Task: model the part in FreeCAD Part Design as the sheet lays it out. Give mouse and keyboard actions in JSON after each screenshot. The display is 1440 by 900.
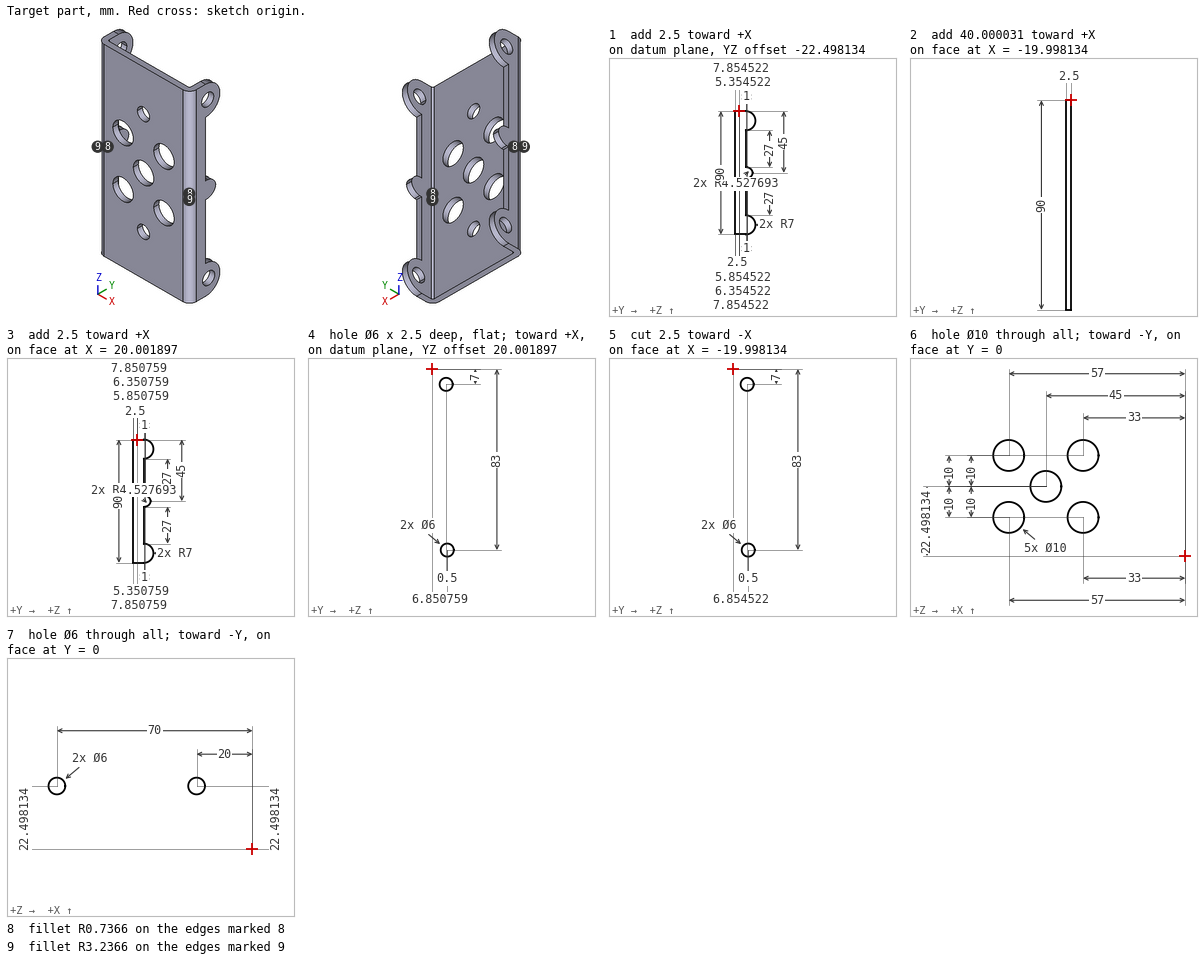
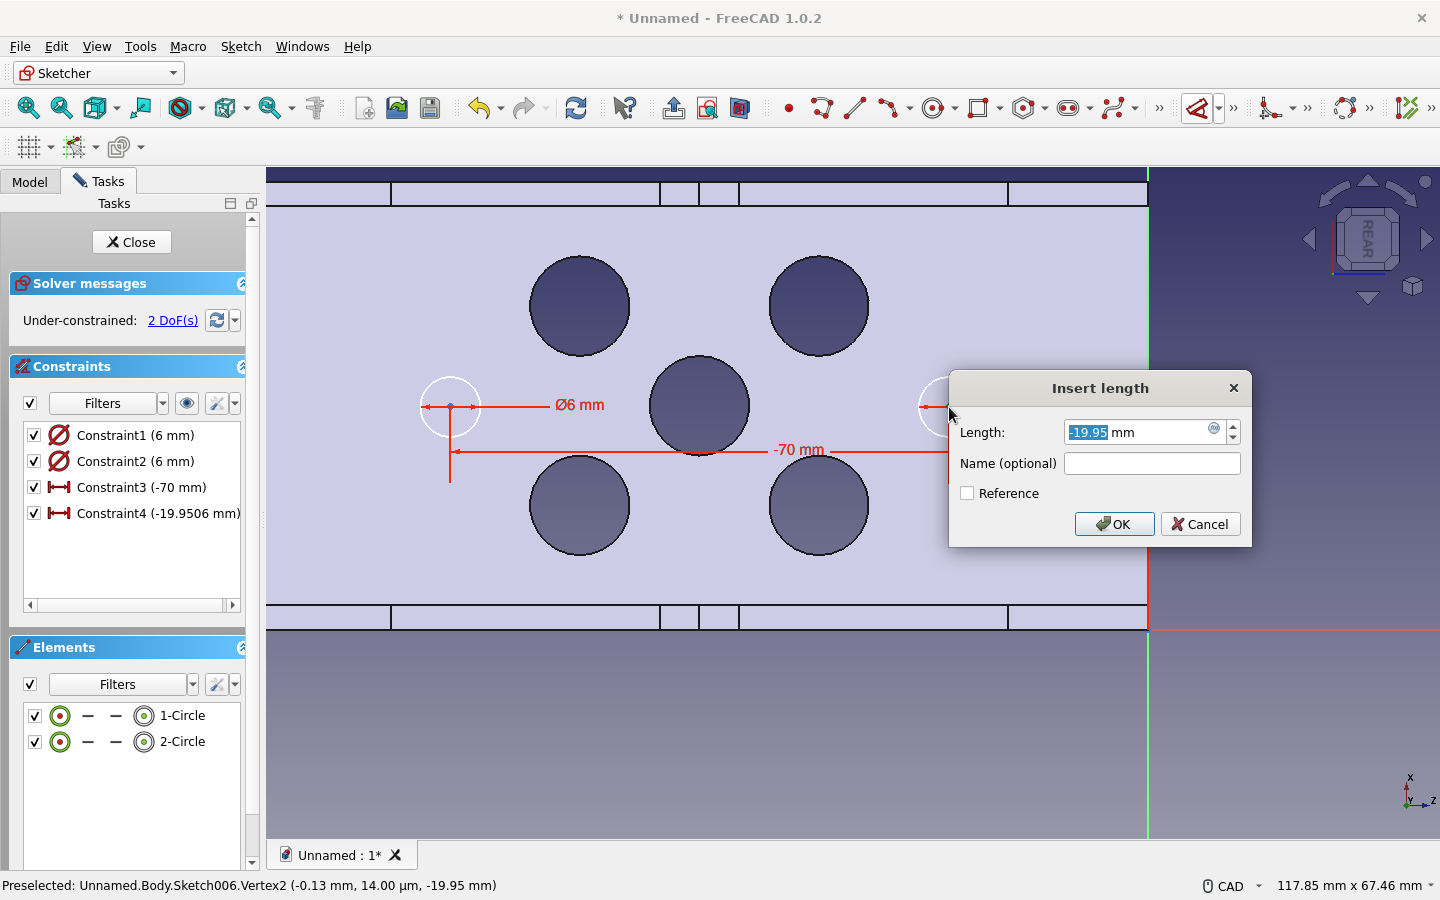
{"action": "type", "text": "-20"}
{"action": "key", "text": "Return"}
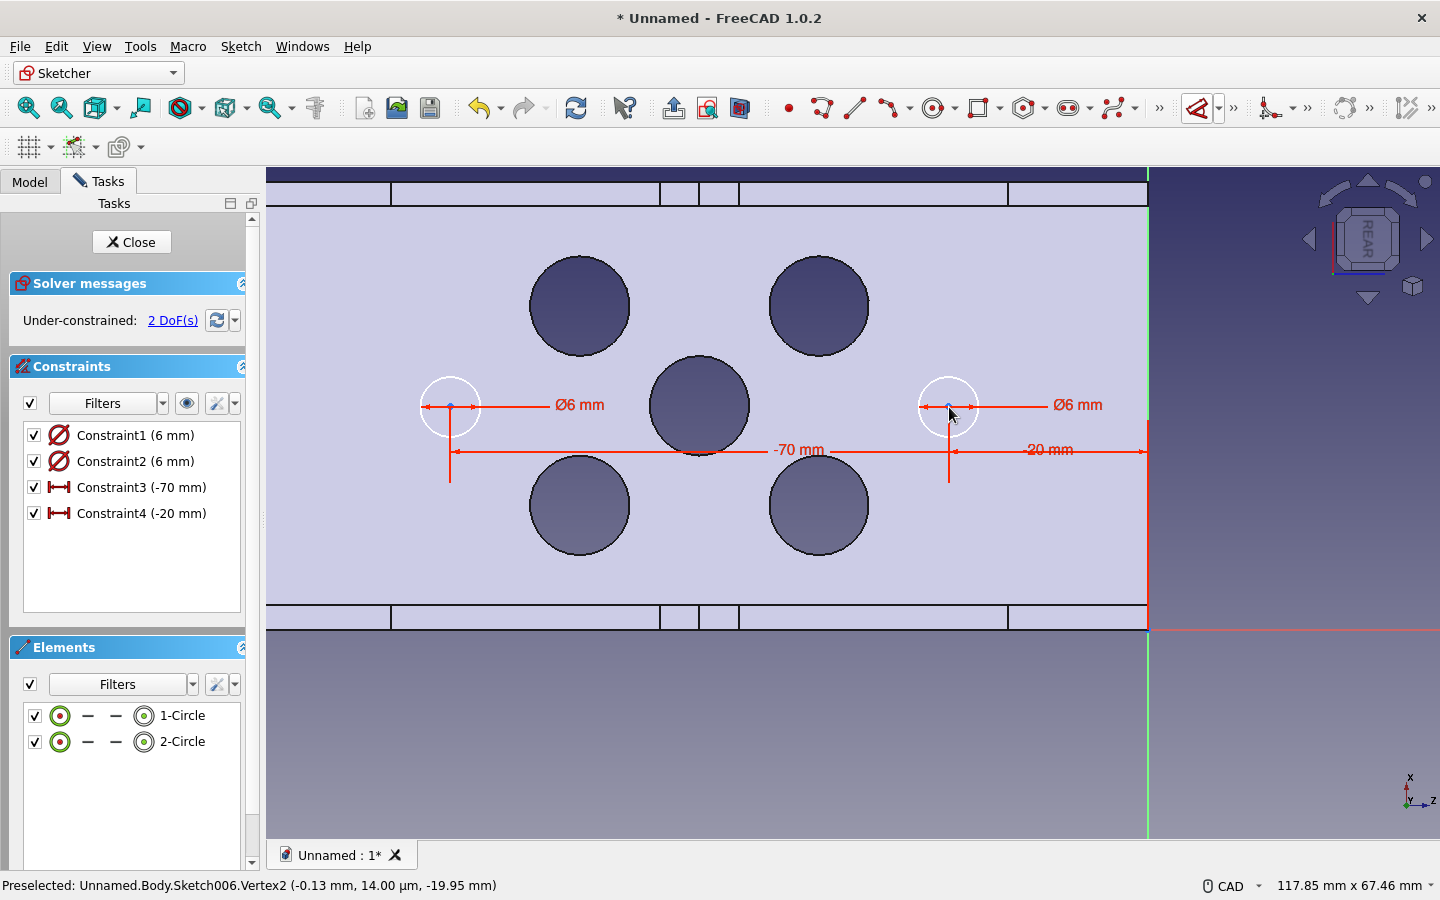
{"action": "left_click", "coordinate": [450, 407]}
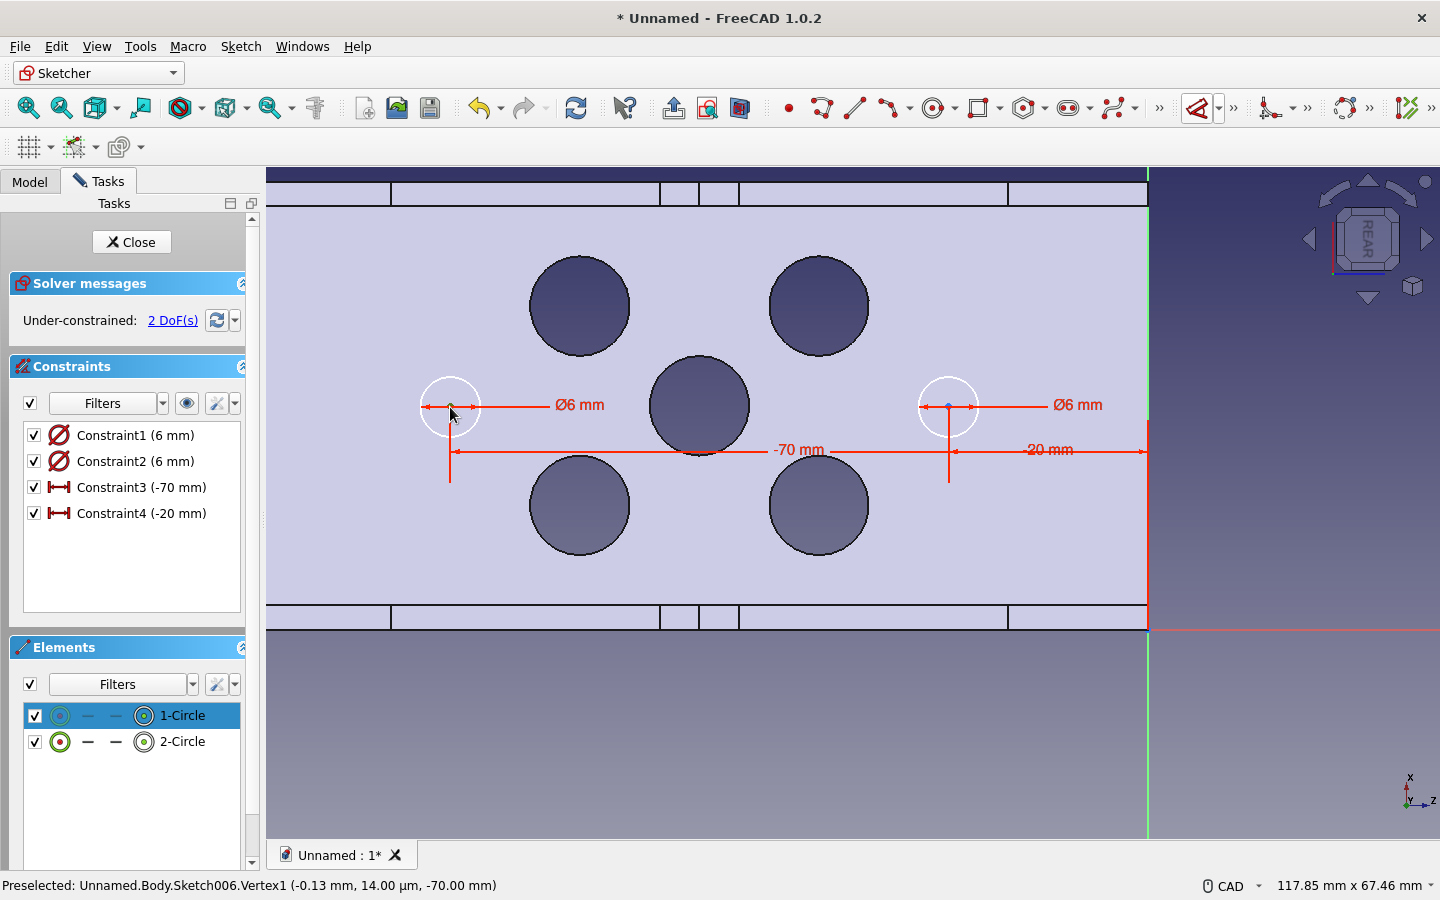
{"action": "left_click", "coordinate": [1218, 108]}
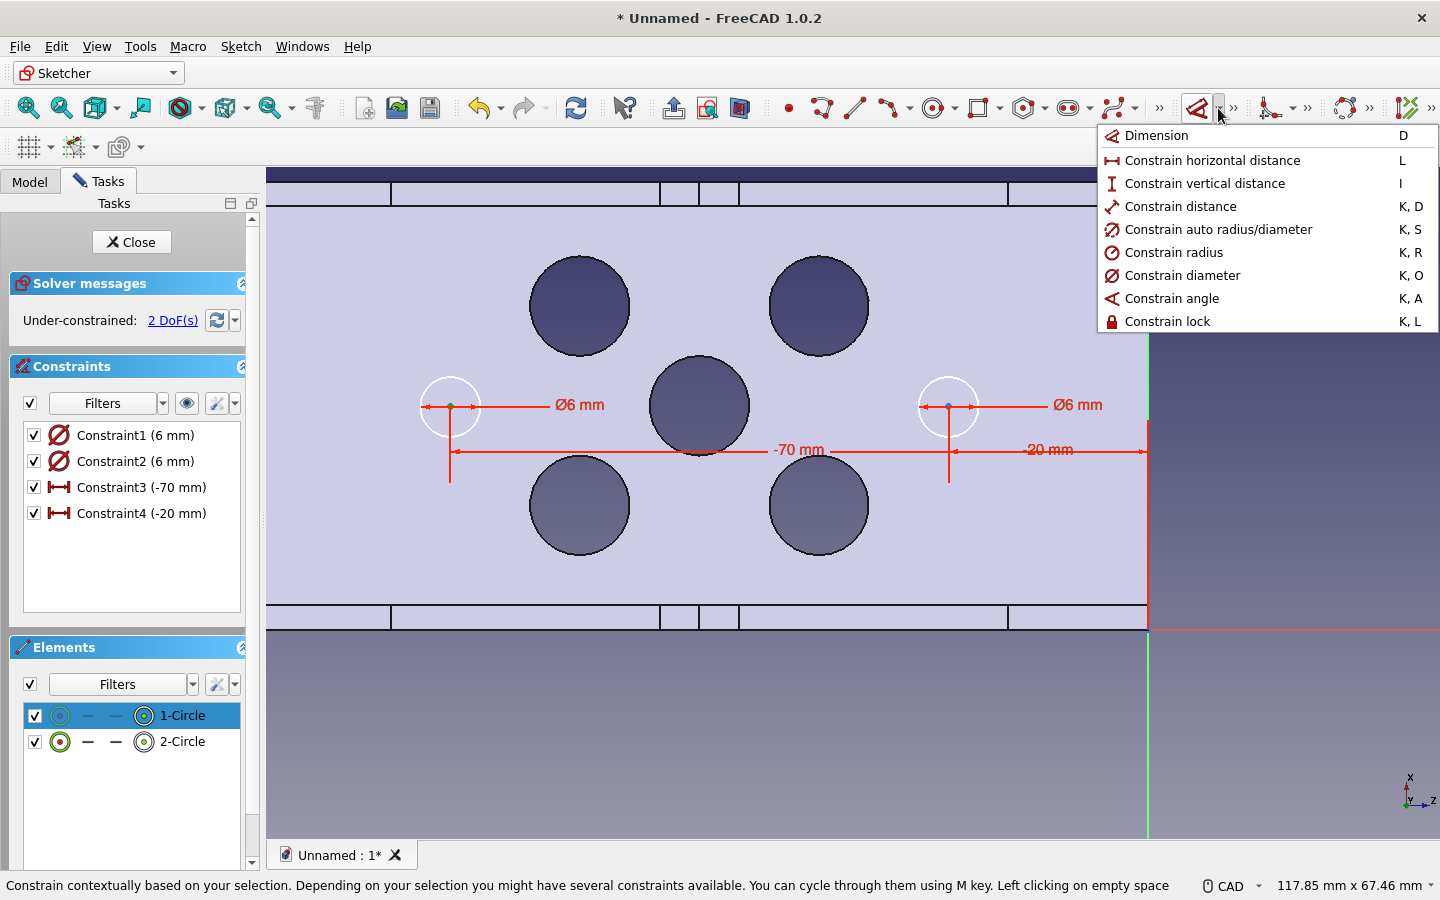
{"action": "left_click", "coordinate": [1268, 184]}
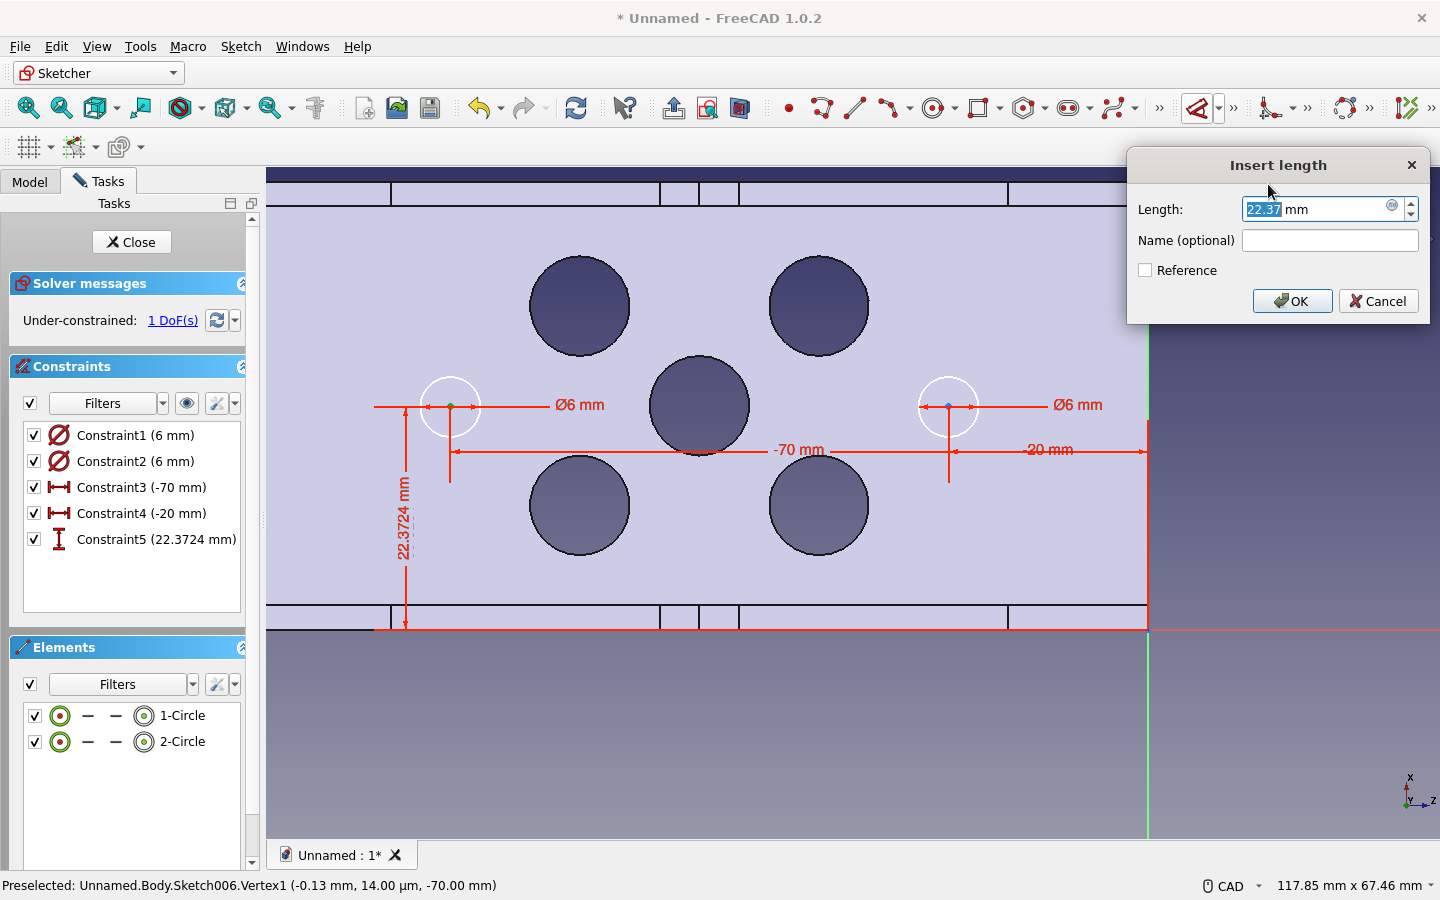
{"action": "type", "text": "22.498134"}
{"action": "key", "text": "Return"}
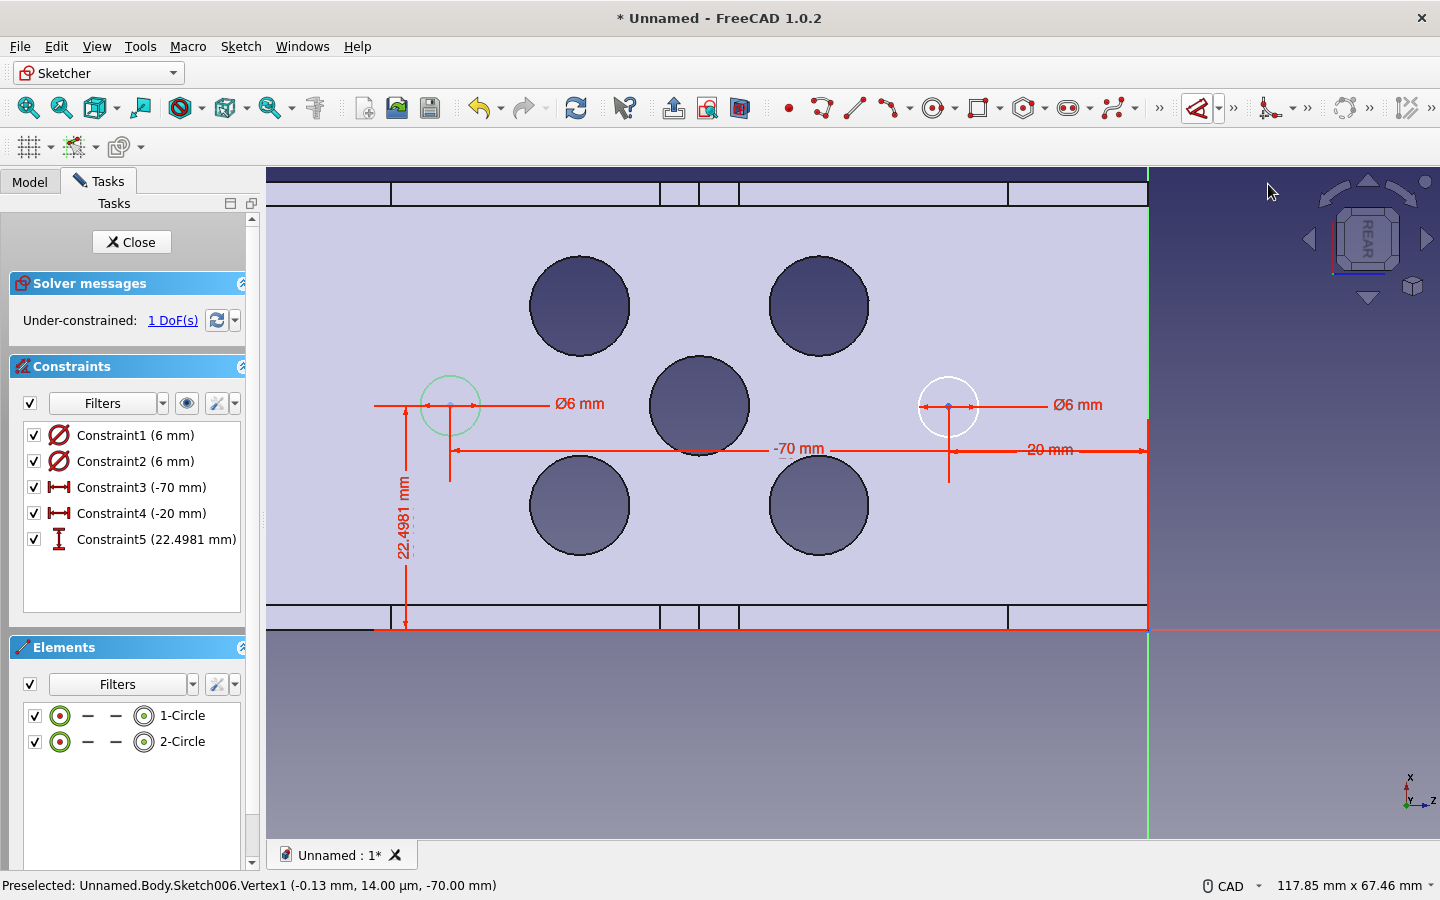
{"action": "left_click", "coordinate": [949, 407]}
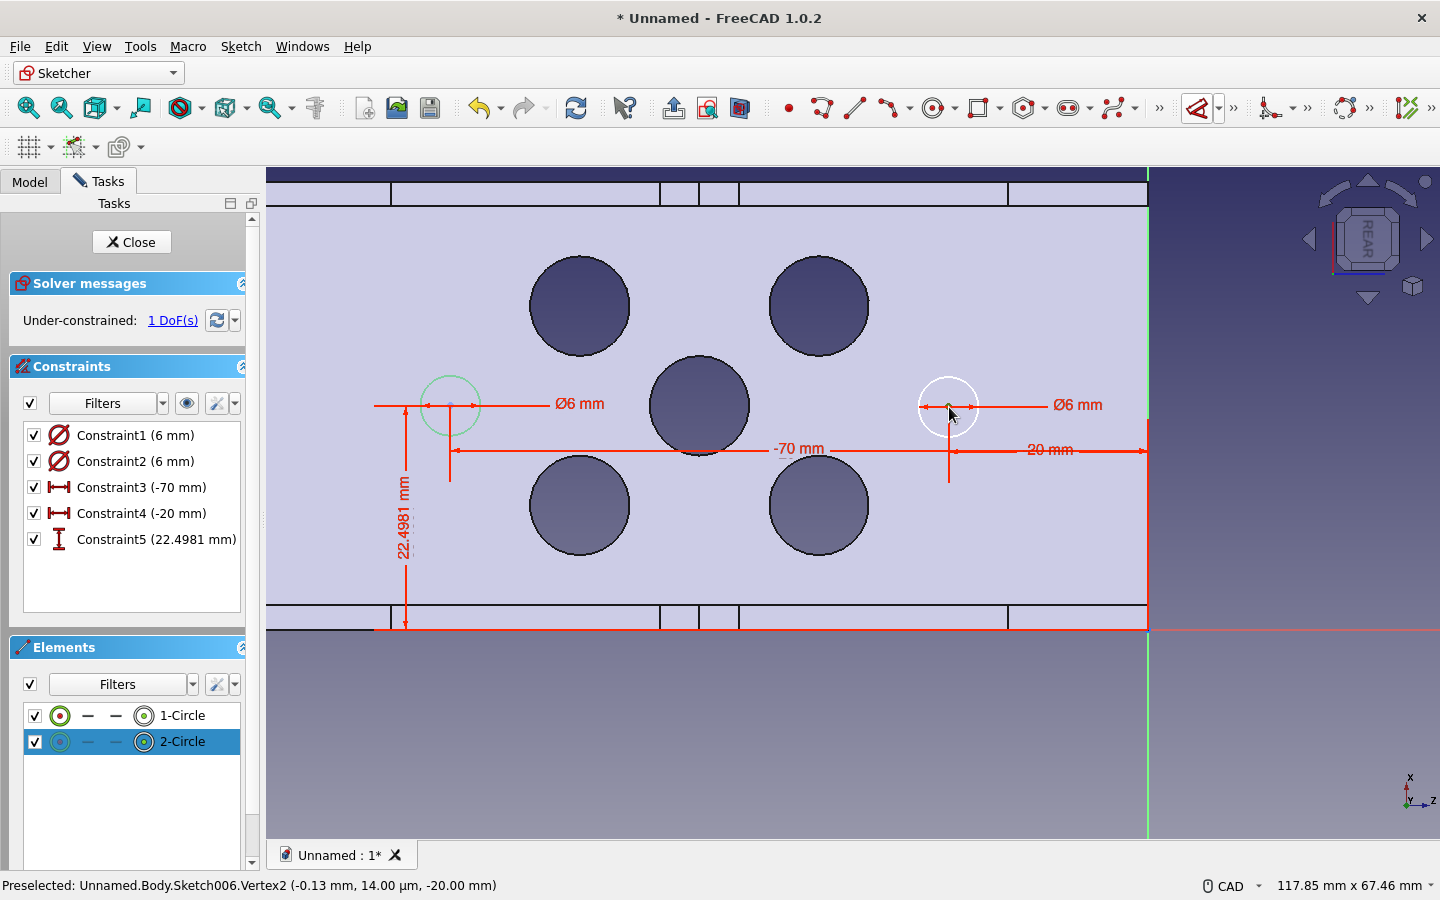
{"action": "key", "text": "i"}